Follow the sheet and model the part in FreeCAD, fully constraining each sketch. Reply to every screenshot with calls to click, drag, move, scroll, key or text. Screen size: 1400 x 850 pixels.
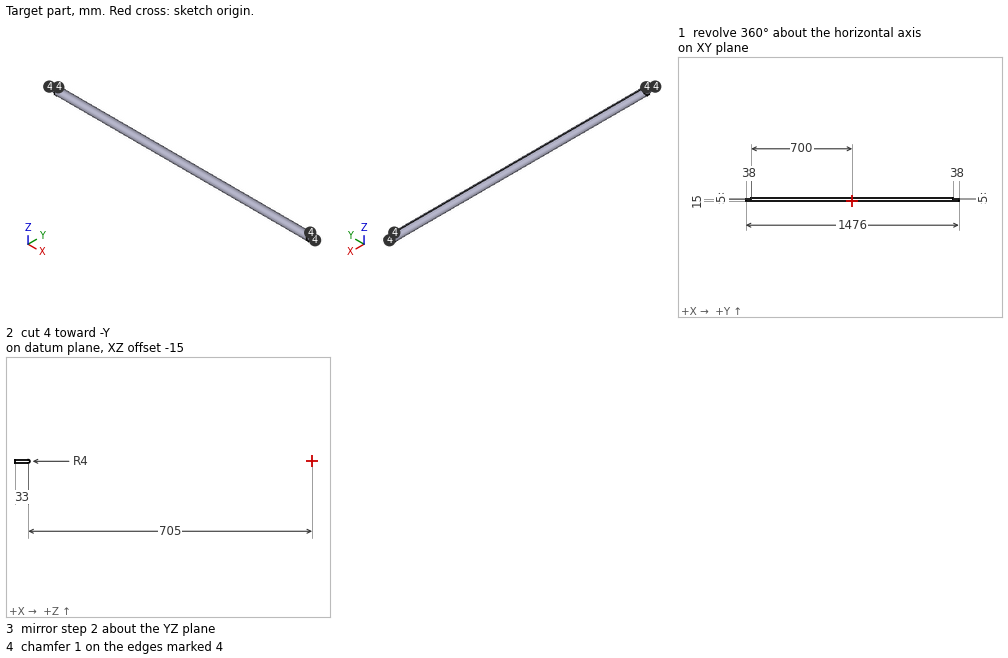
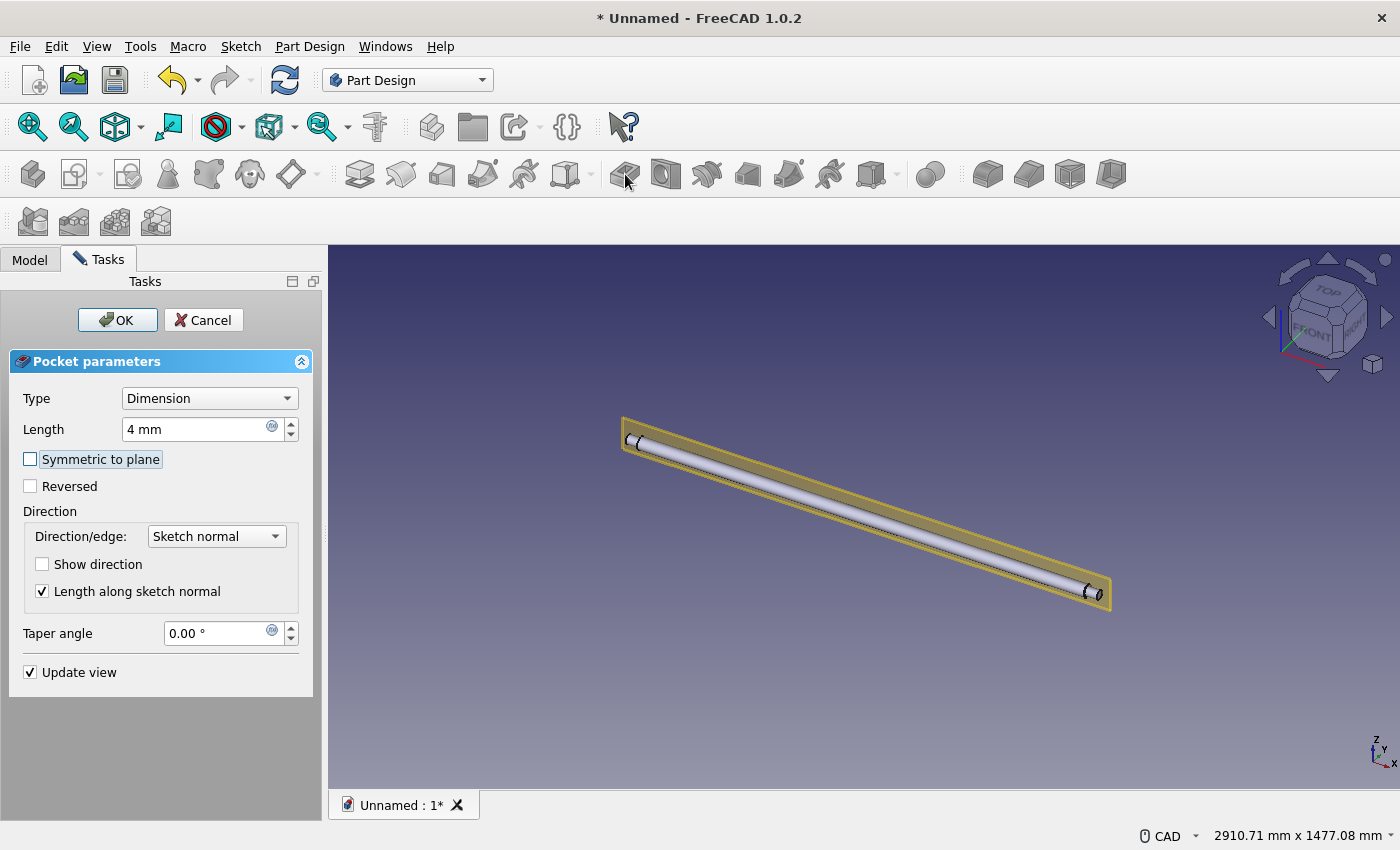
click(31, 486)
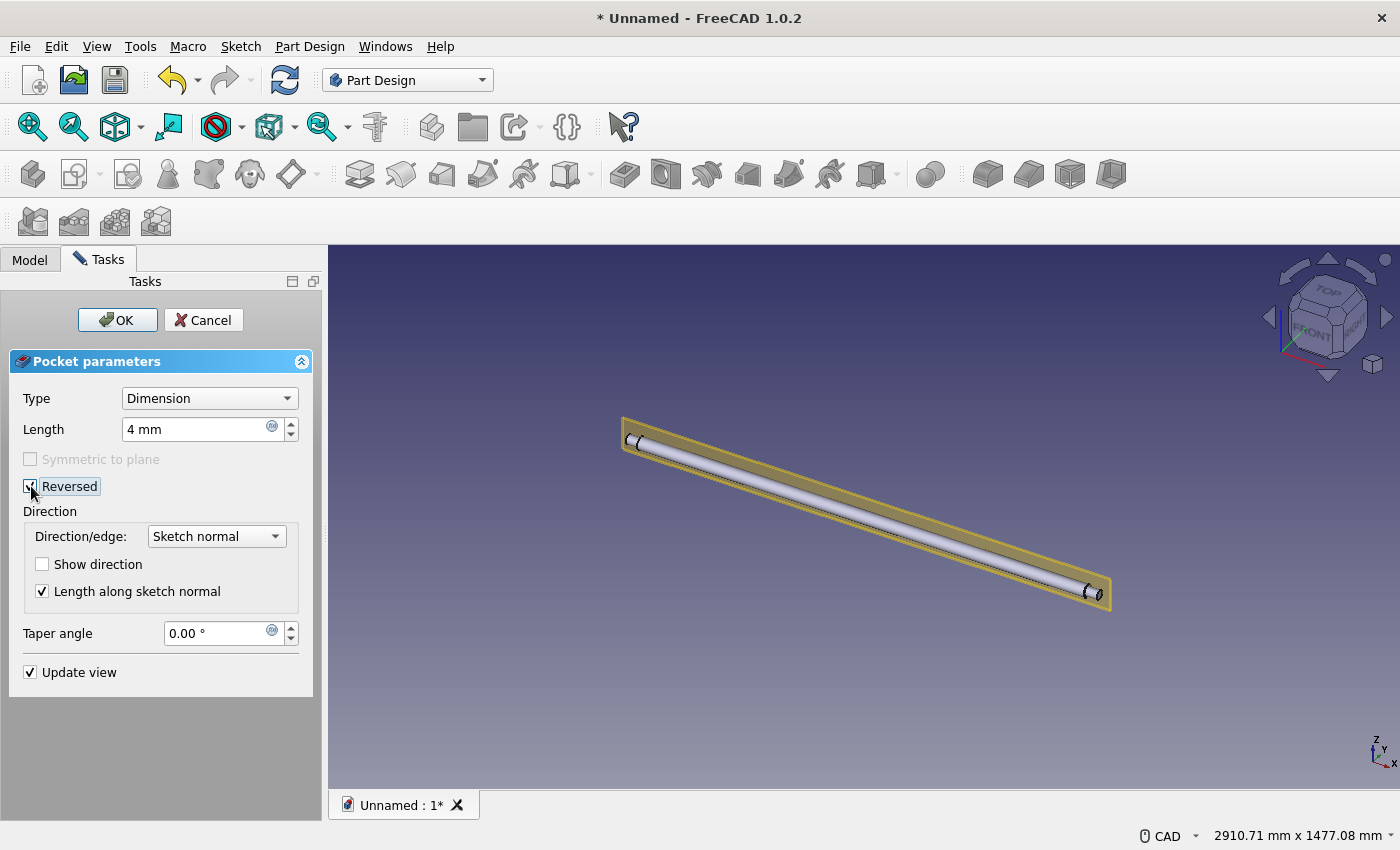
click(118, 320)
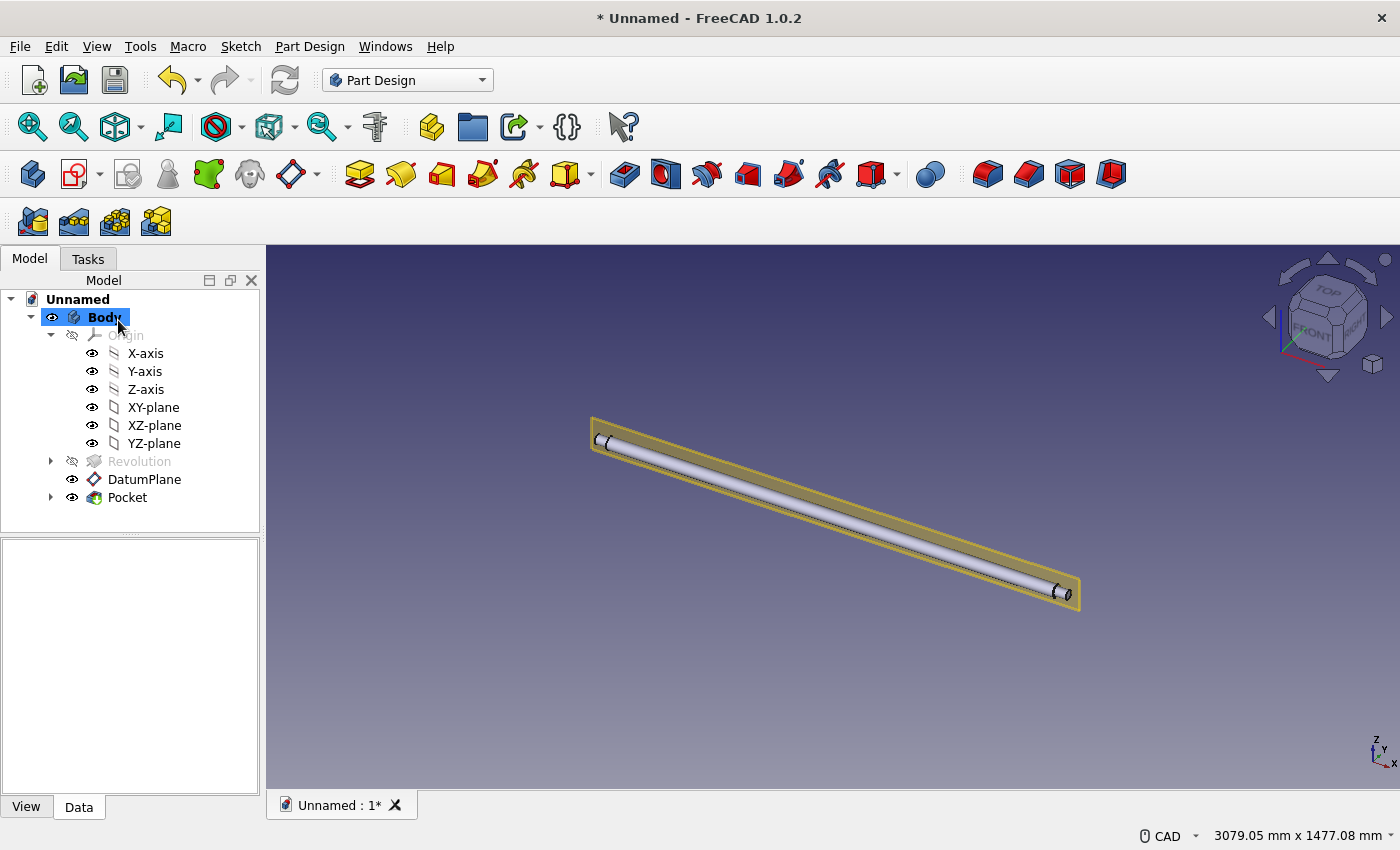
click(117, 479)
key(space)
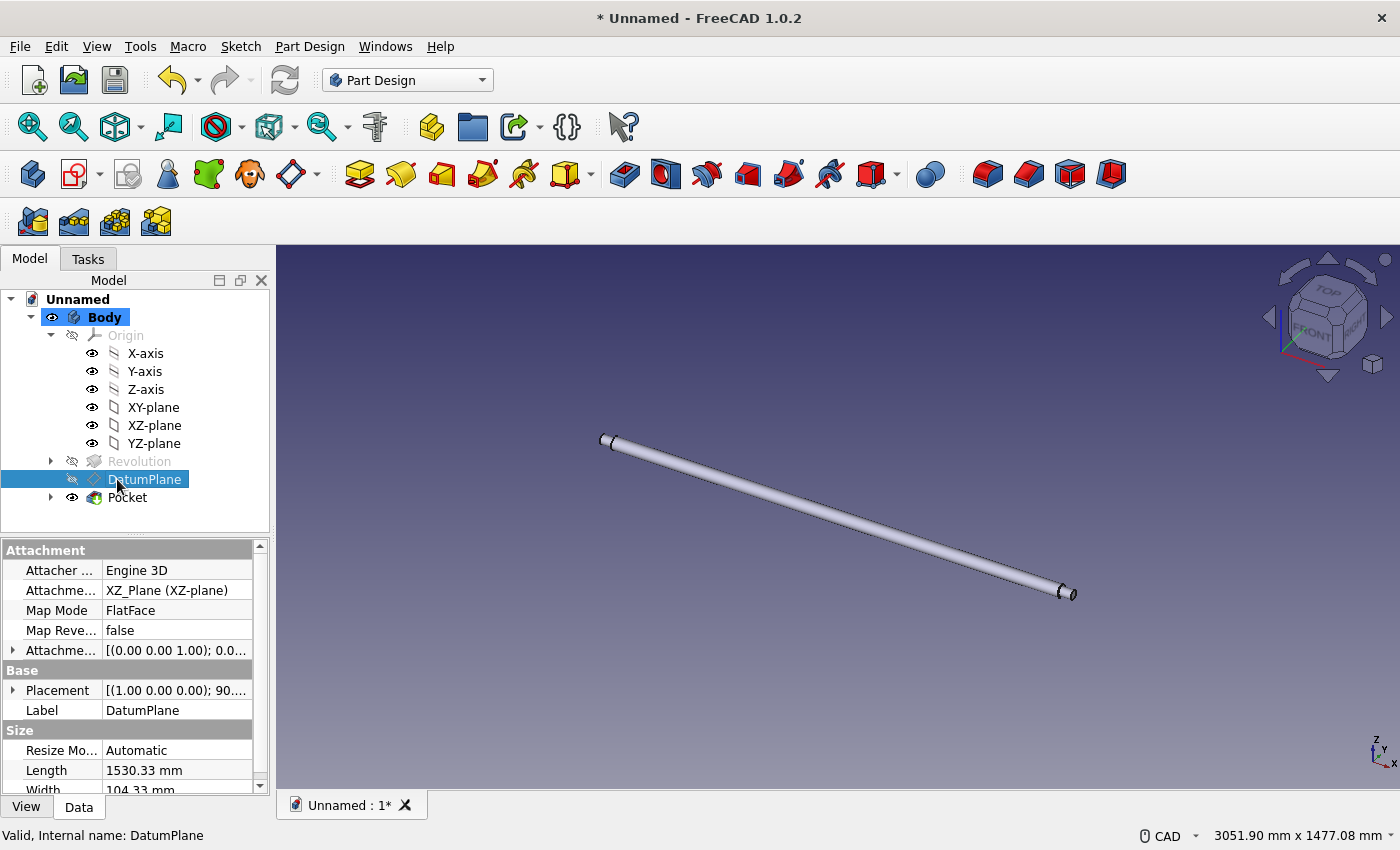
click(33, 128)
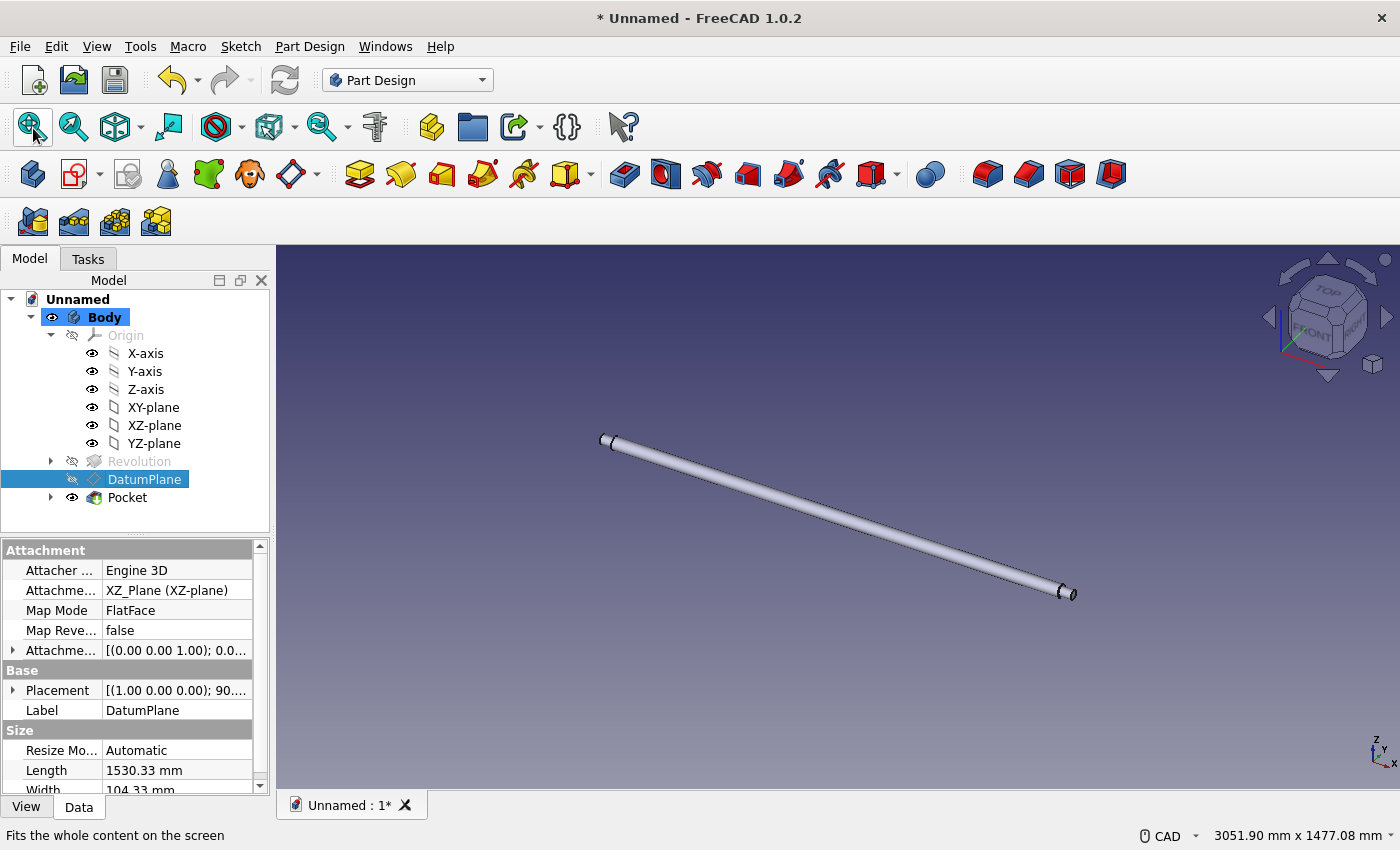
click(117, 497)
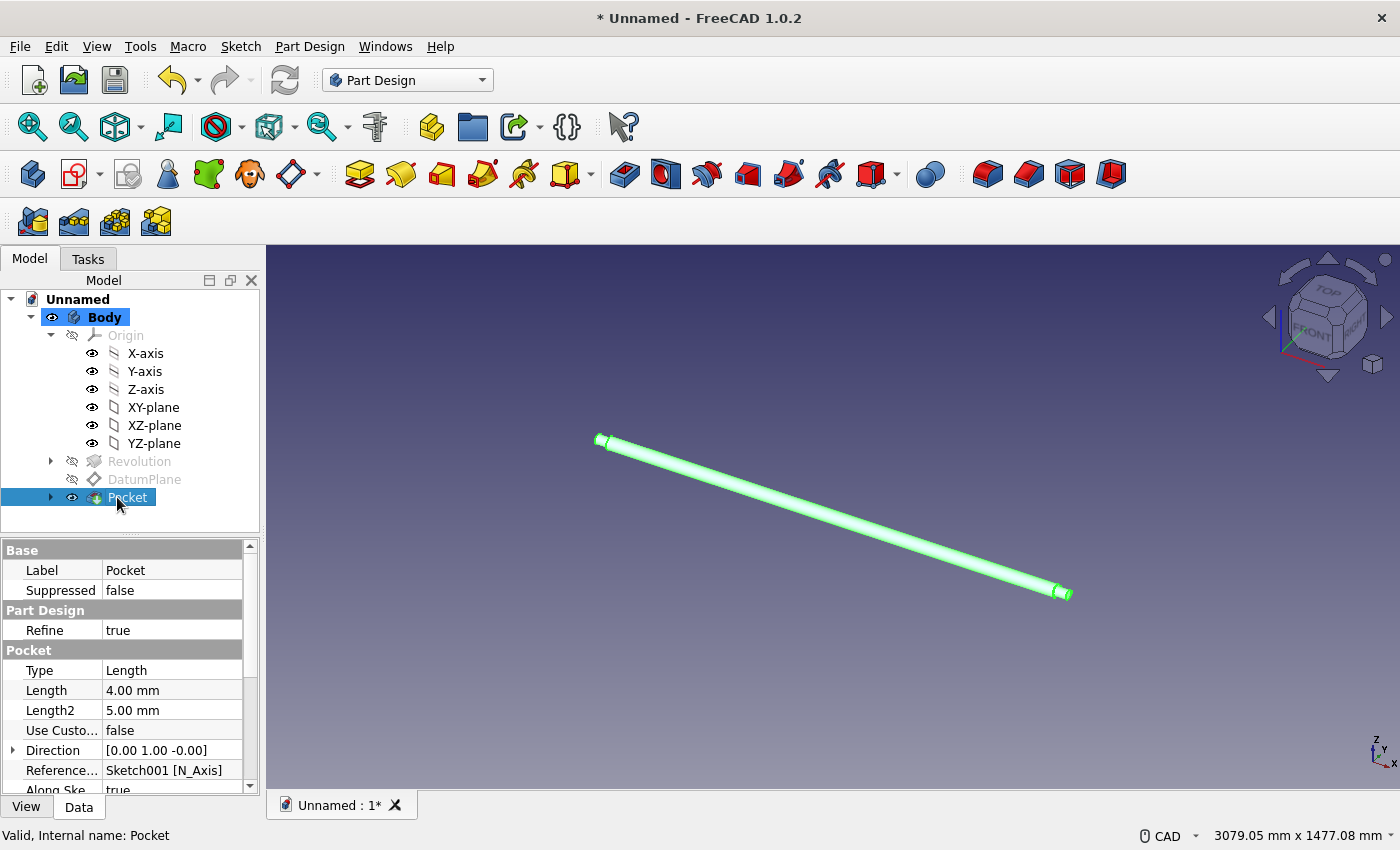
click(33, 222)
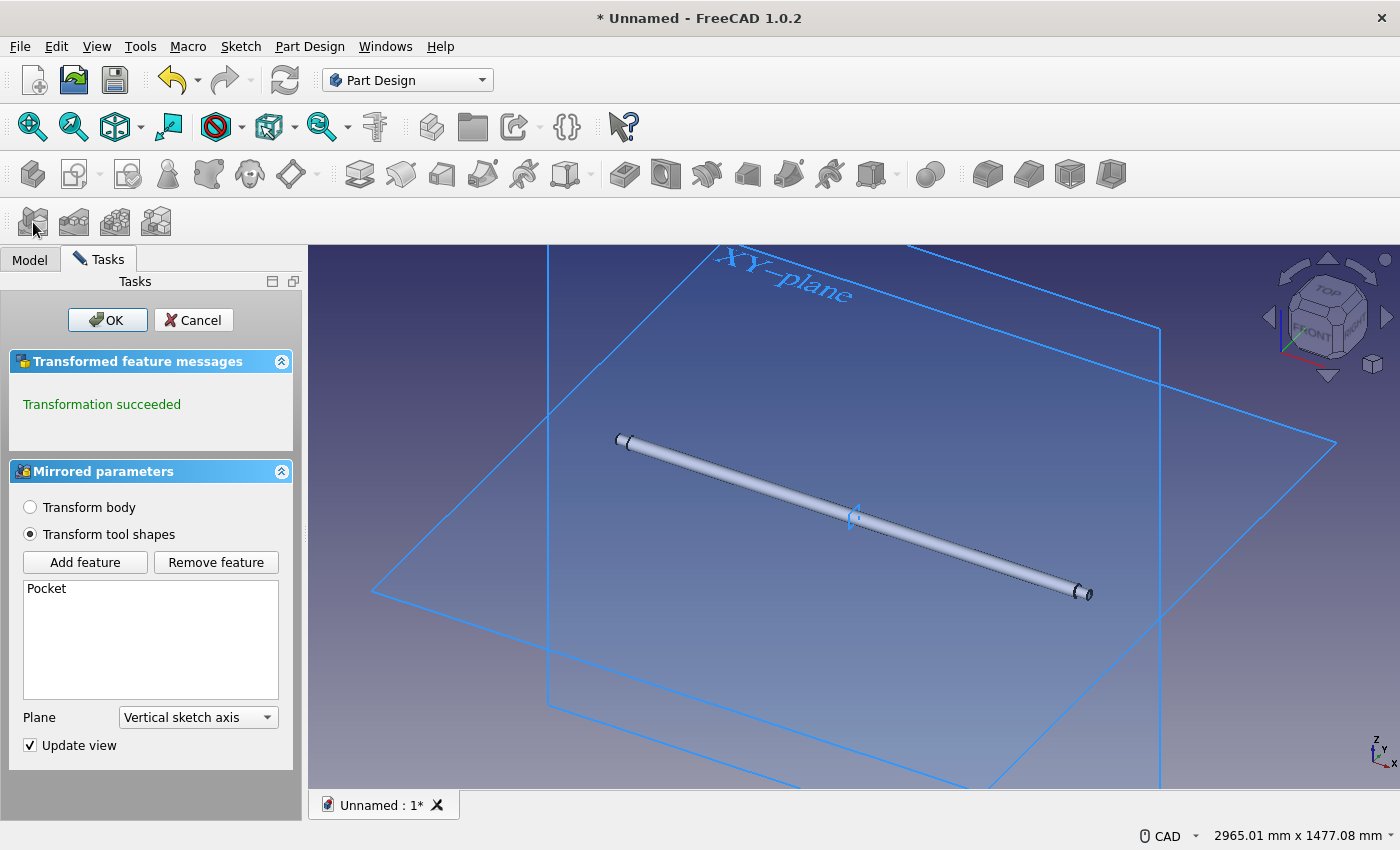
click(199, 718)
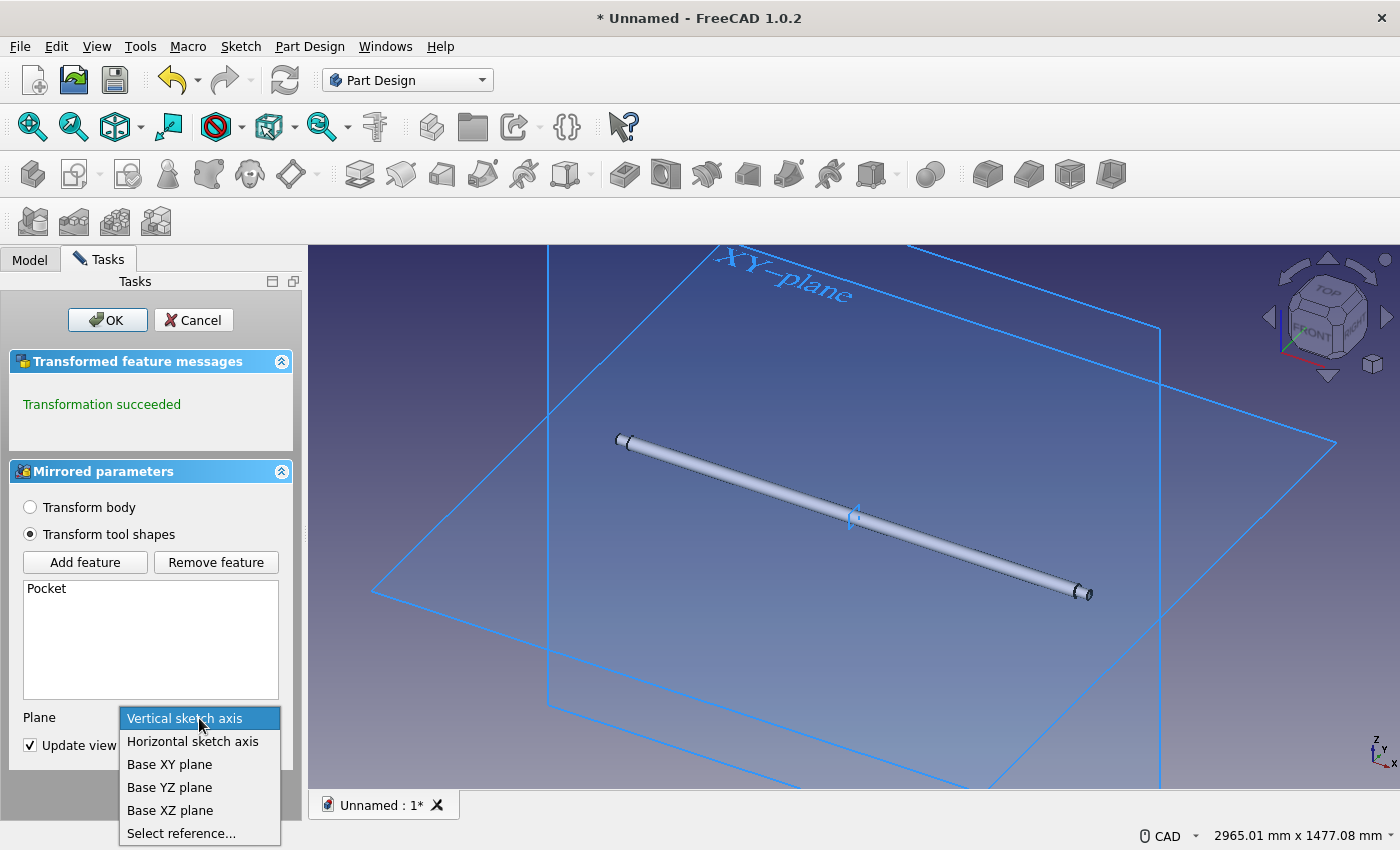
click(198, 788)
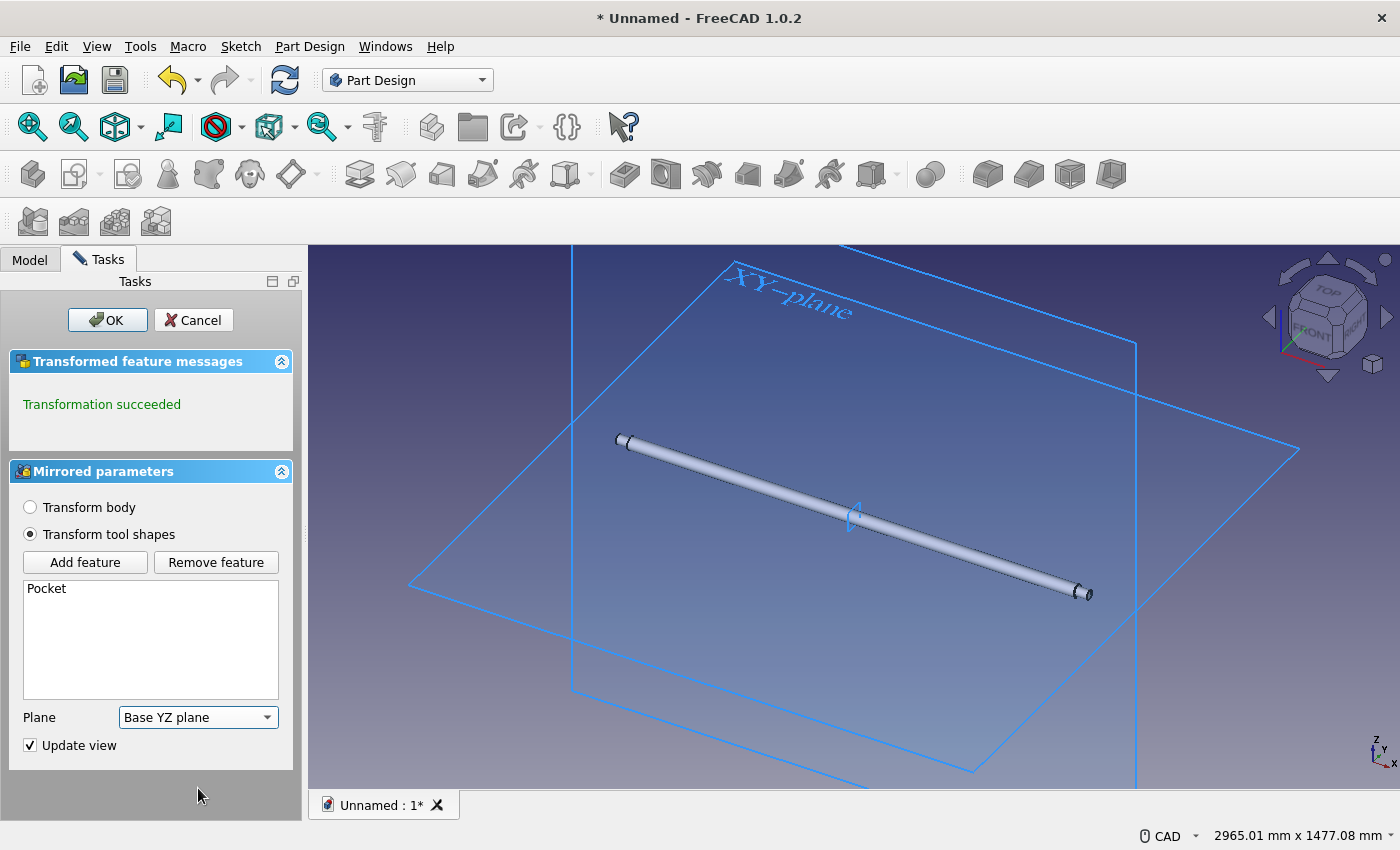
click(108, 320)